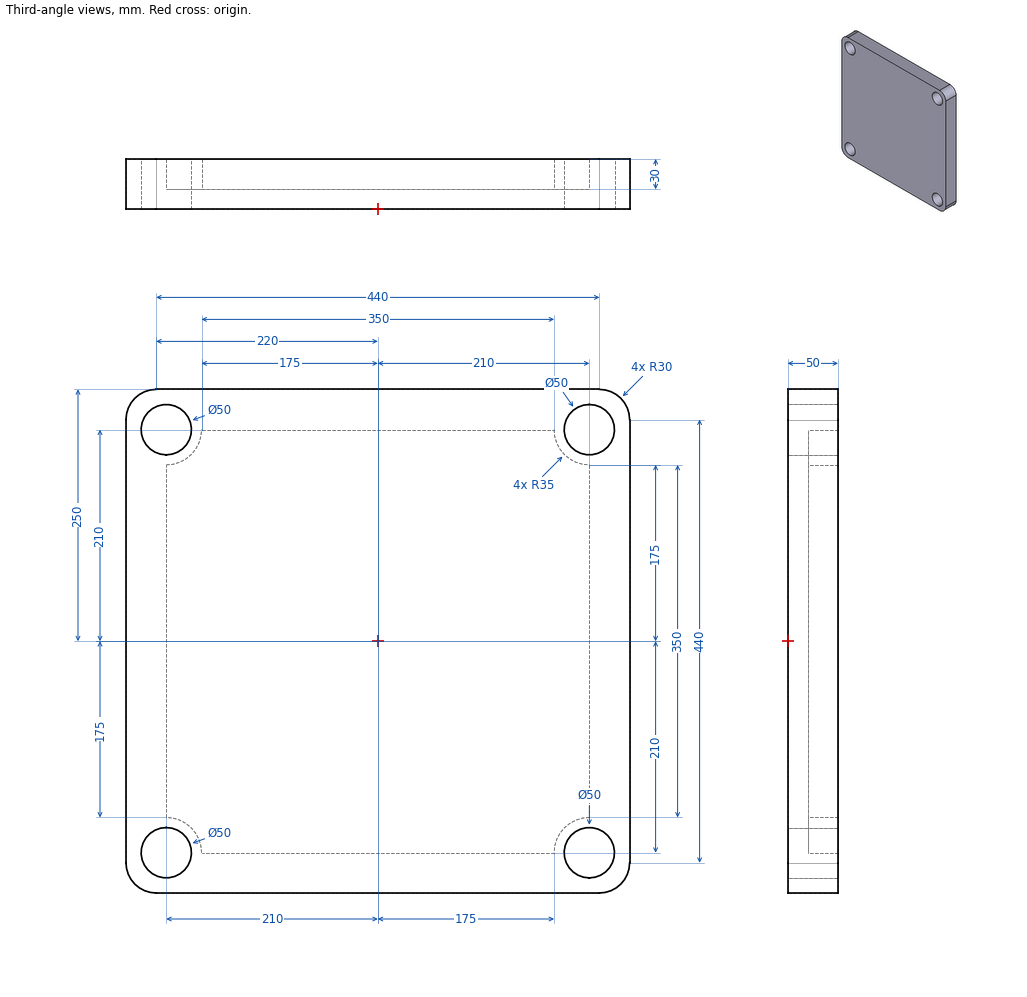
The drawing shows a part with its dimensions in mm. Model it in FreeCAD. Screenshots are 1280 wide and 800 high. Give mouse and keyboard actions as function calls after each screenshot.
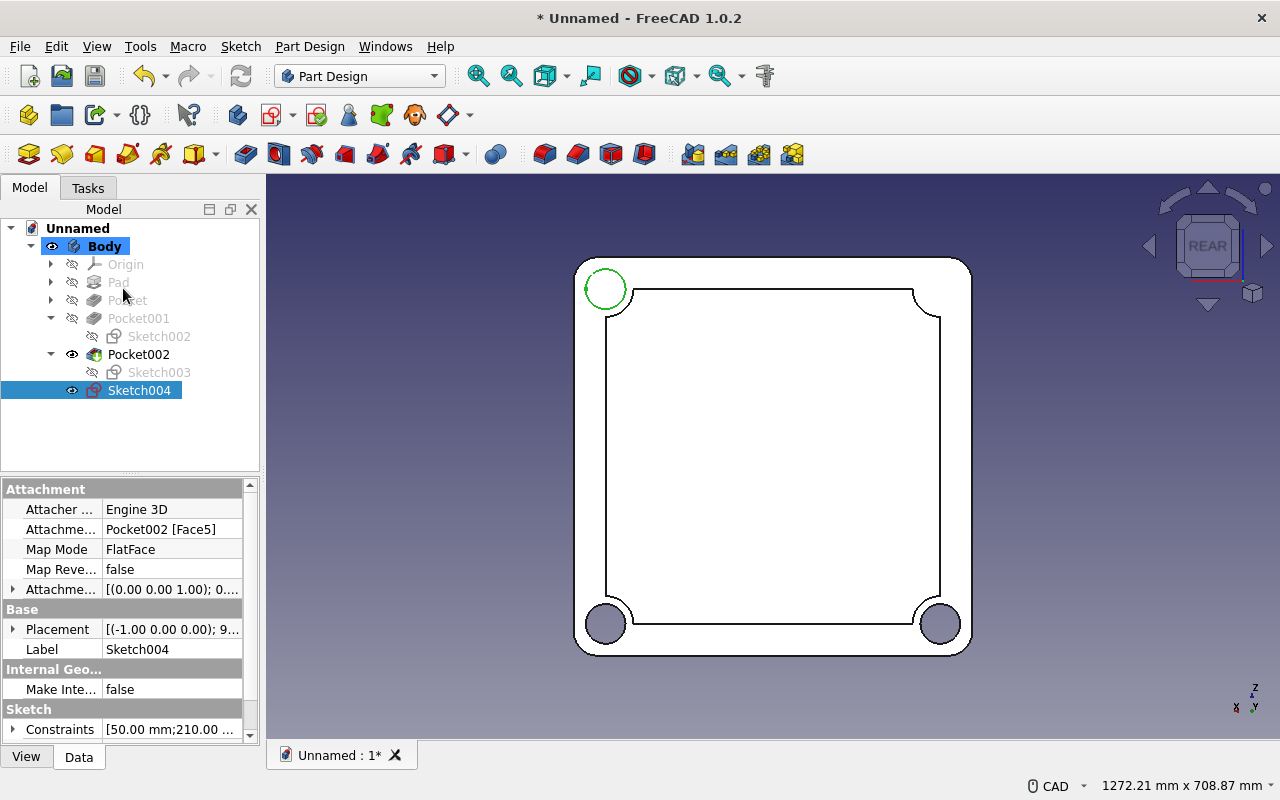
click(246, 154)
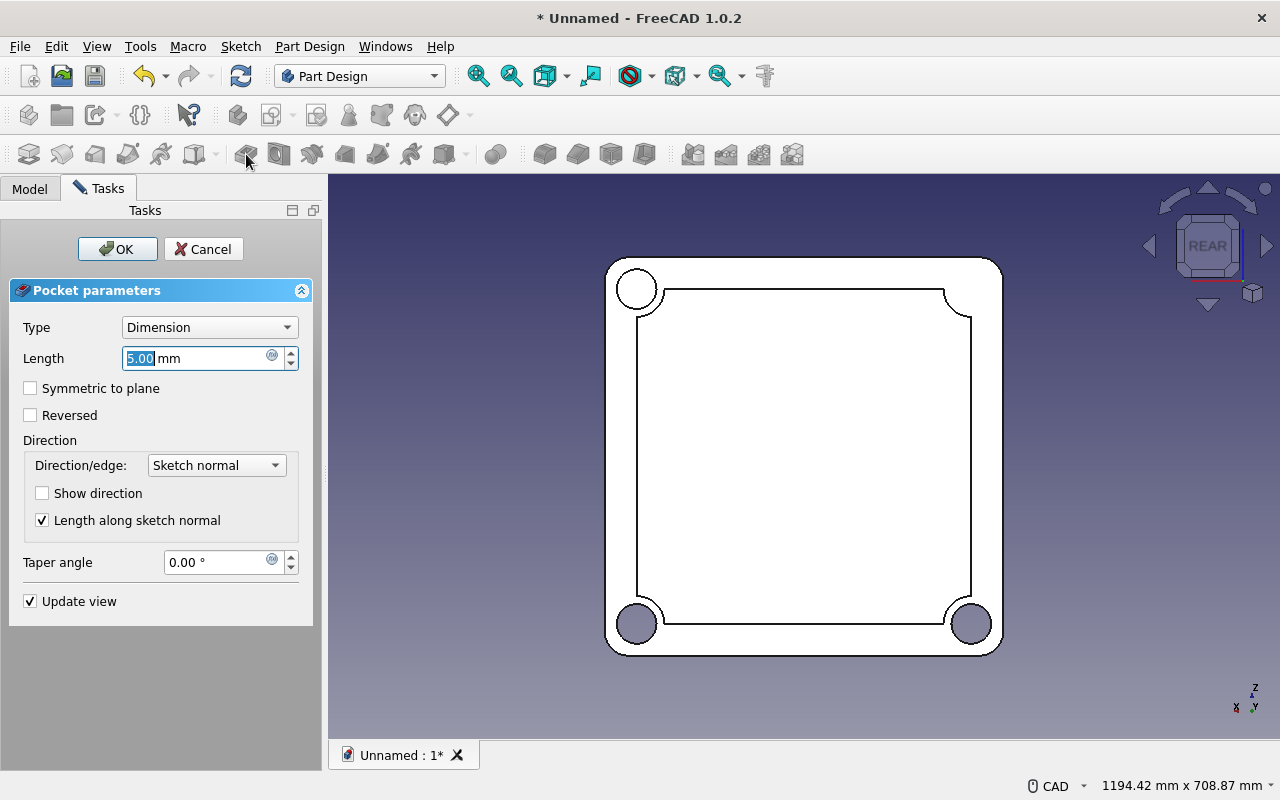
click(210, 328)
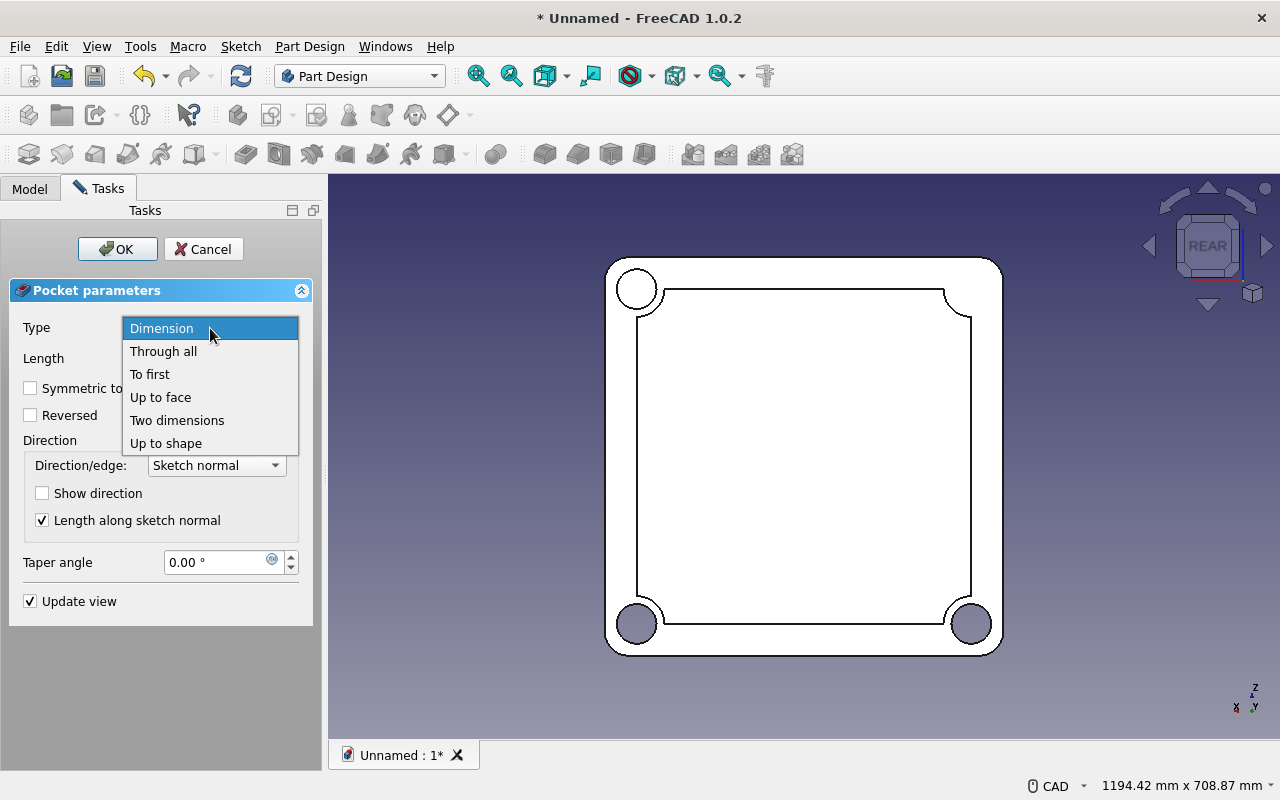
click(208, 374)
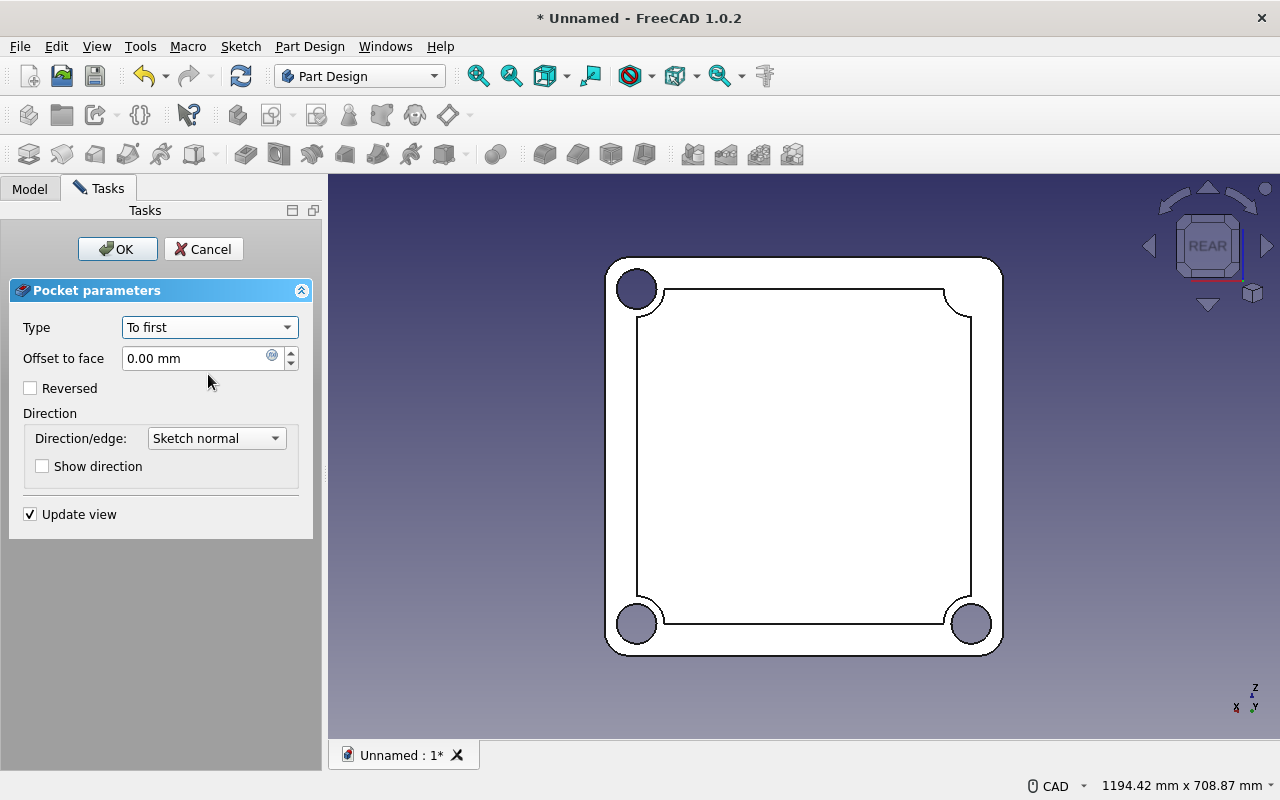
click(118, 249)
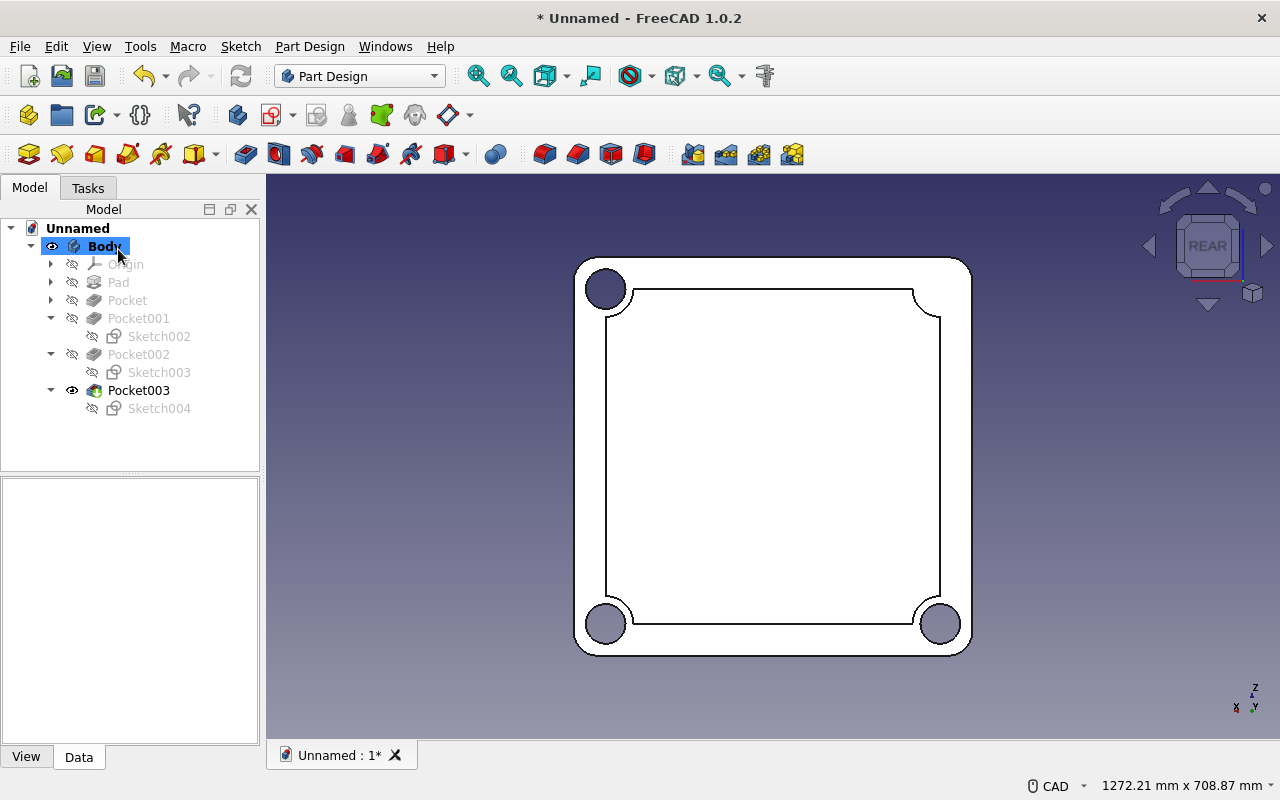
click(944, 285)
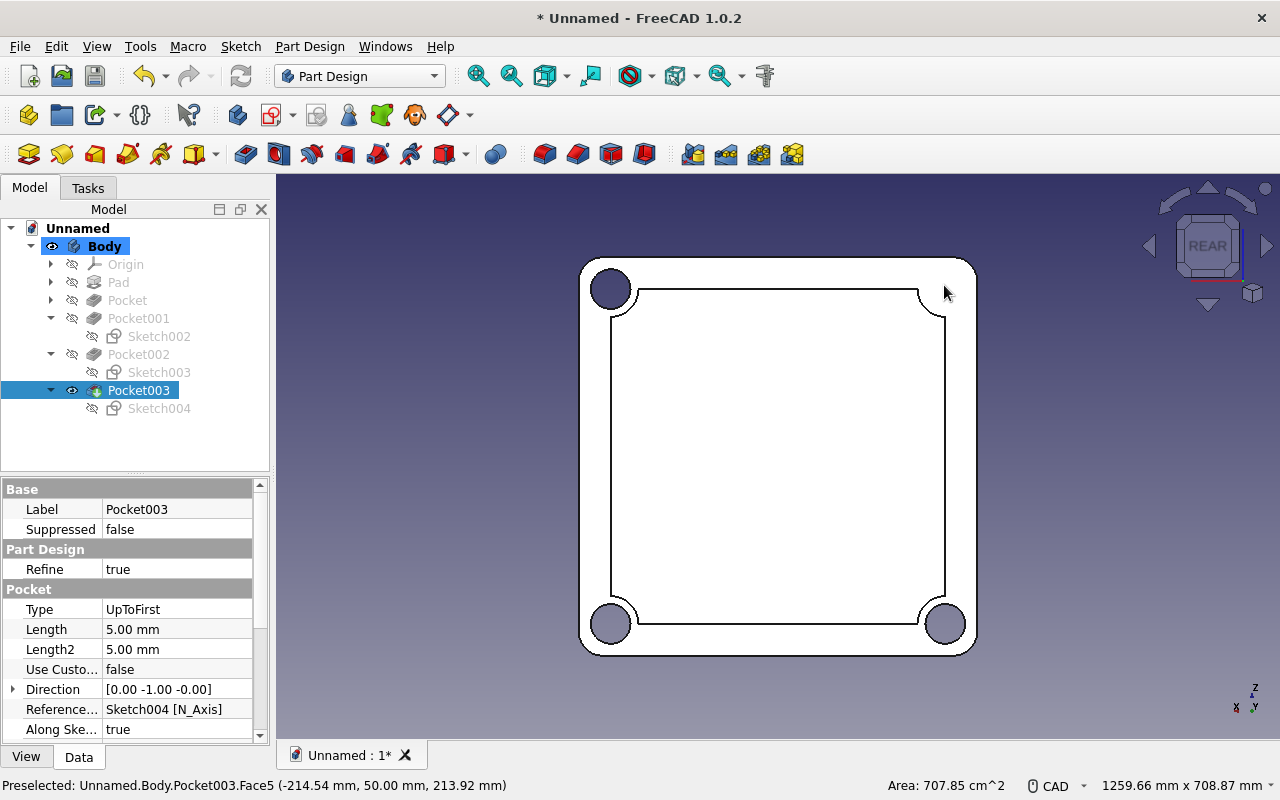
click(270, 116)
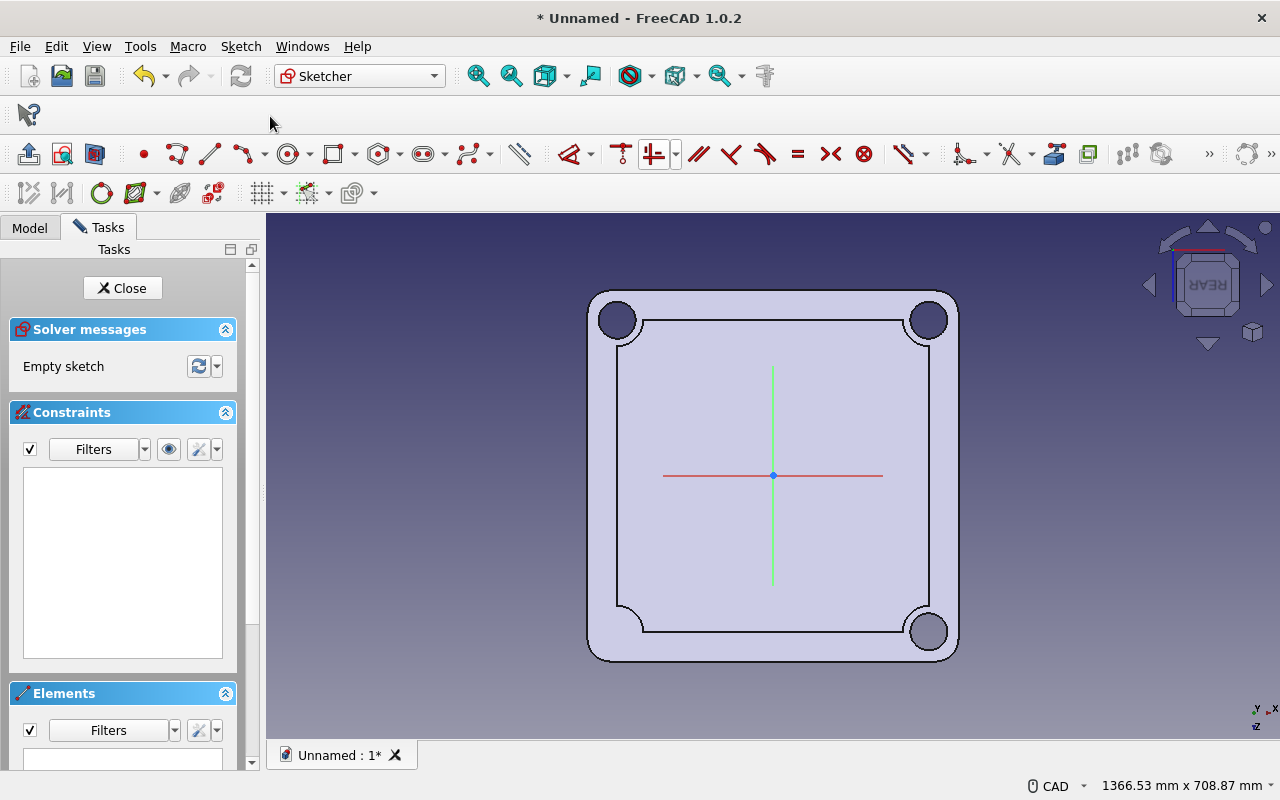
scroll(606, 651, up, 11)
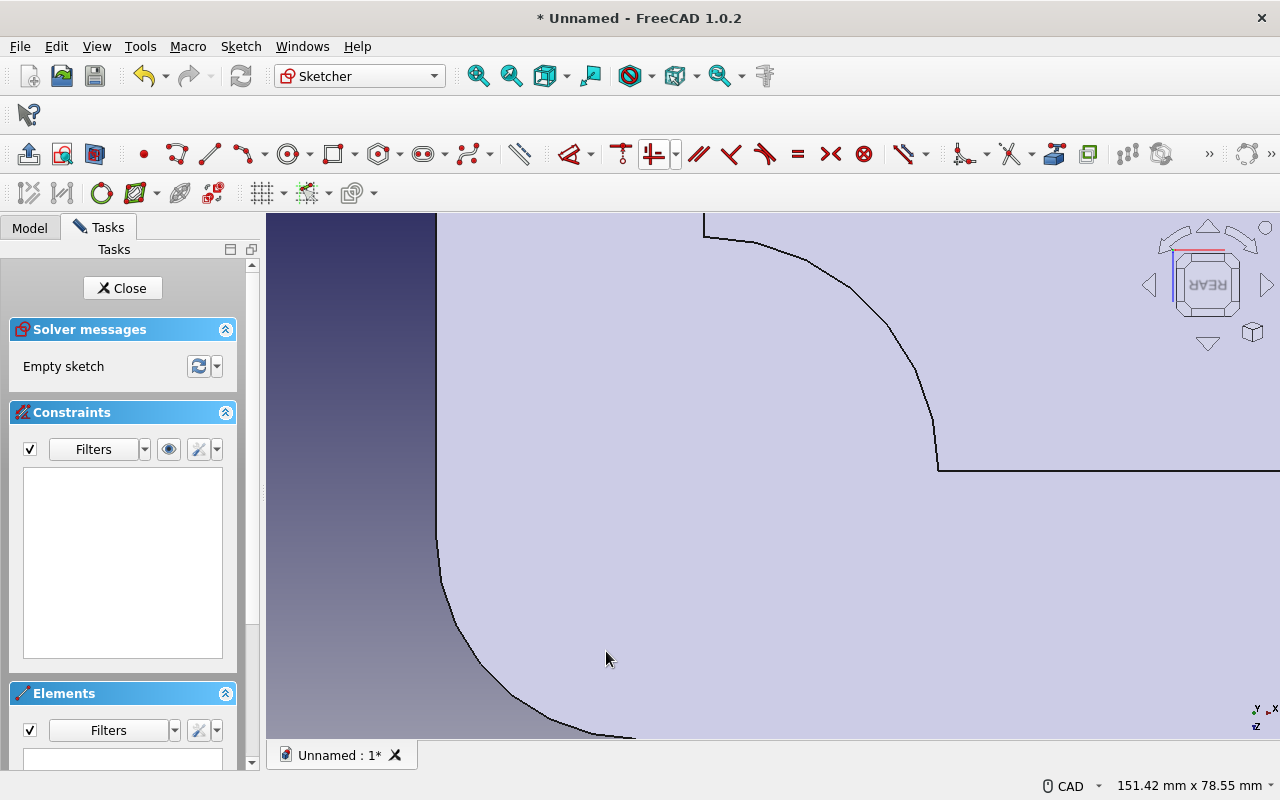
click(288, 154)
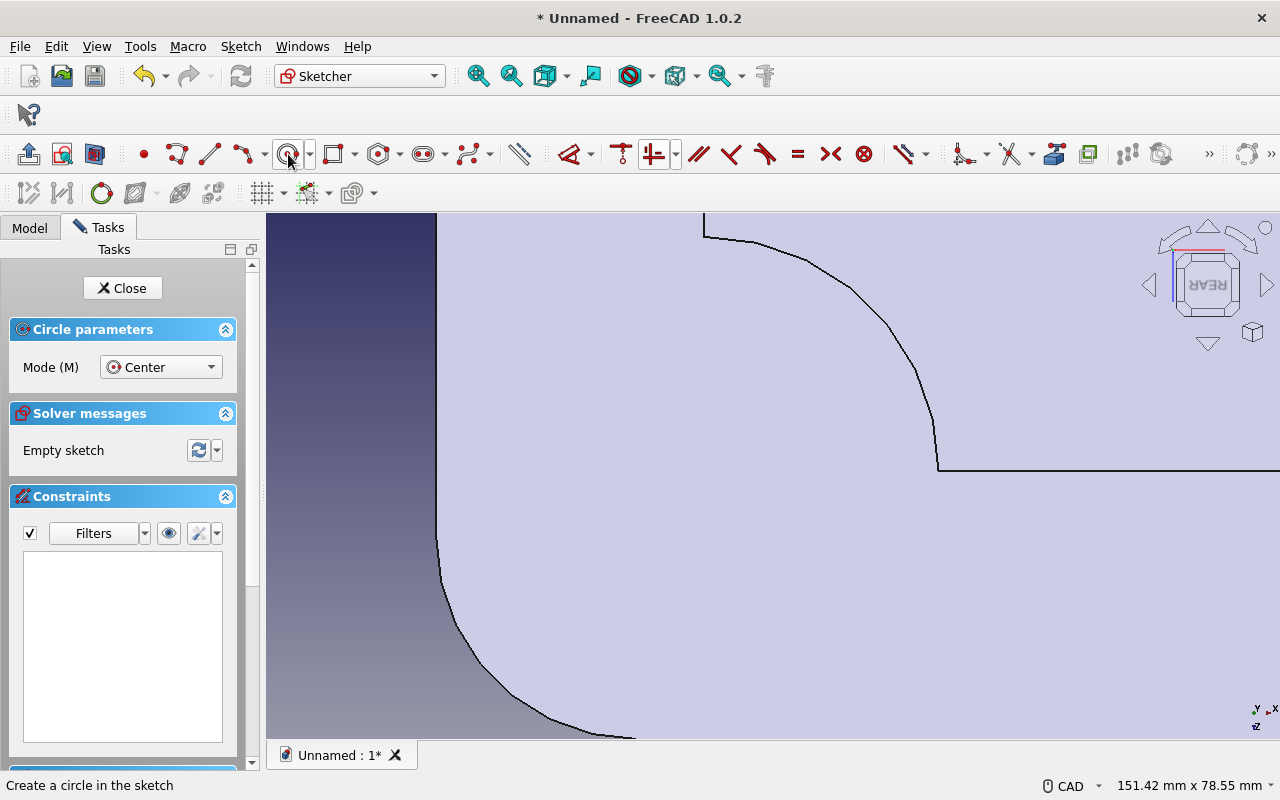
click(704, 471)
move(823, 353)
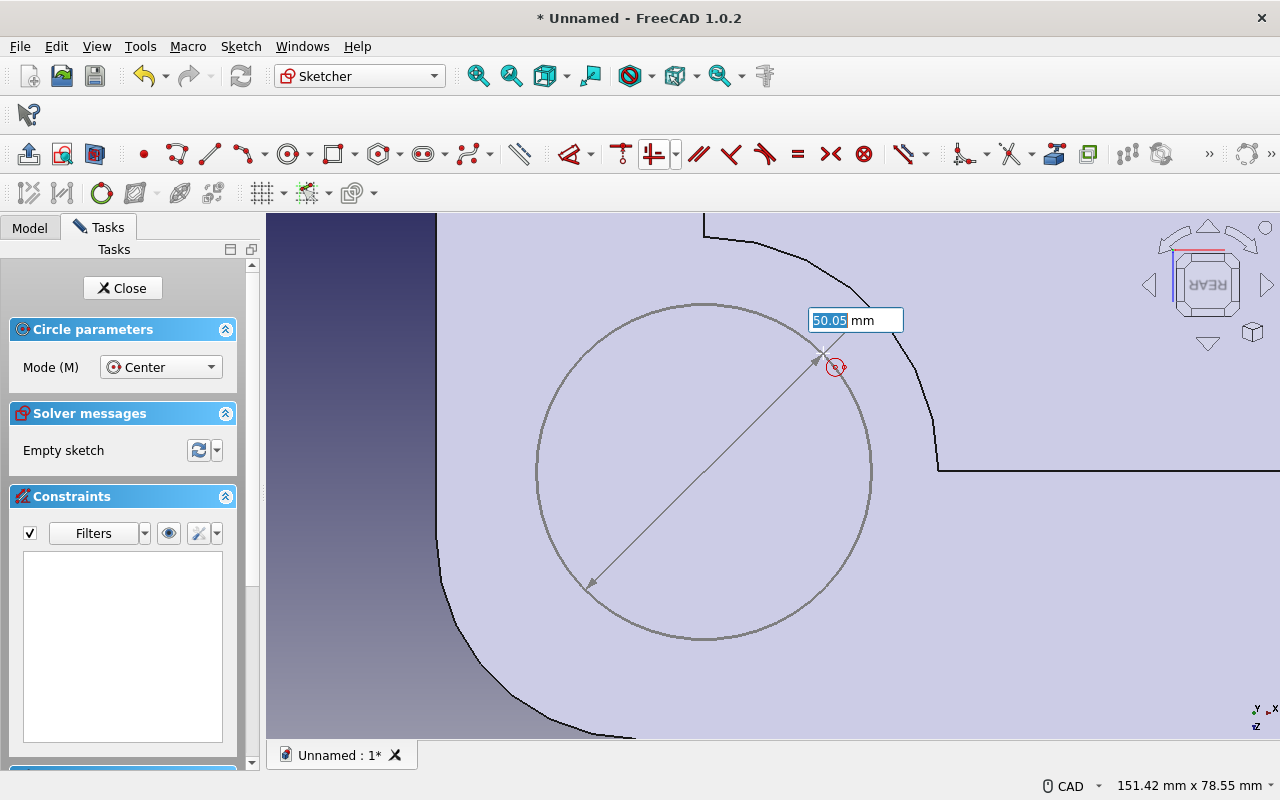
text(50)
key(Return)
key(Escape)